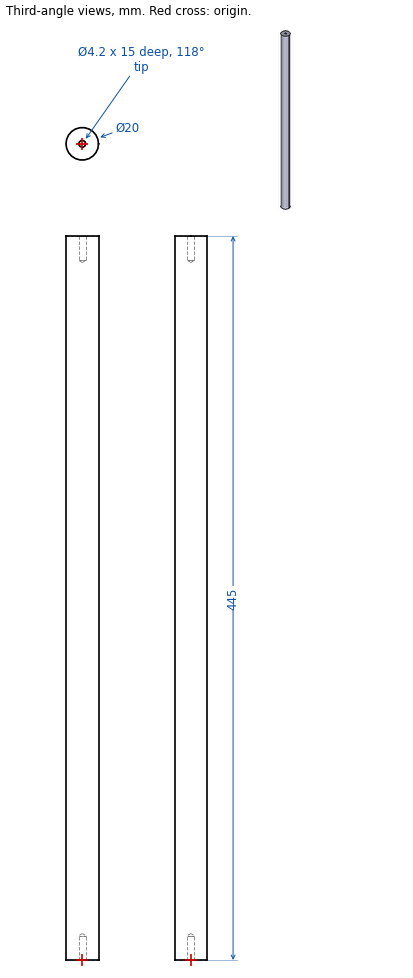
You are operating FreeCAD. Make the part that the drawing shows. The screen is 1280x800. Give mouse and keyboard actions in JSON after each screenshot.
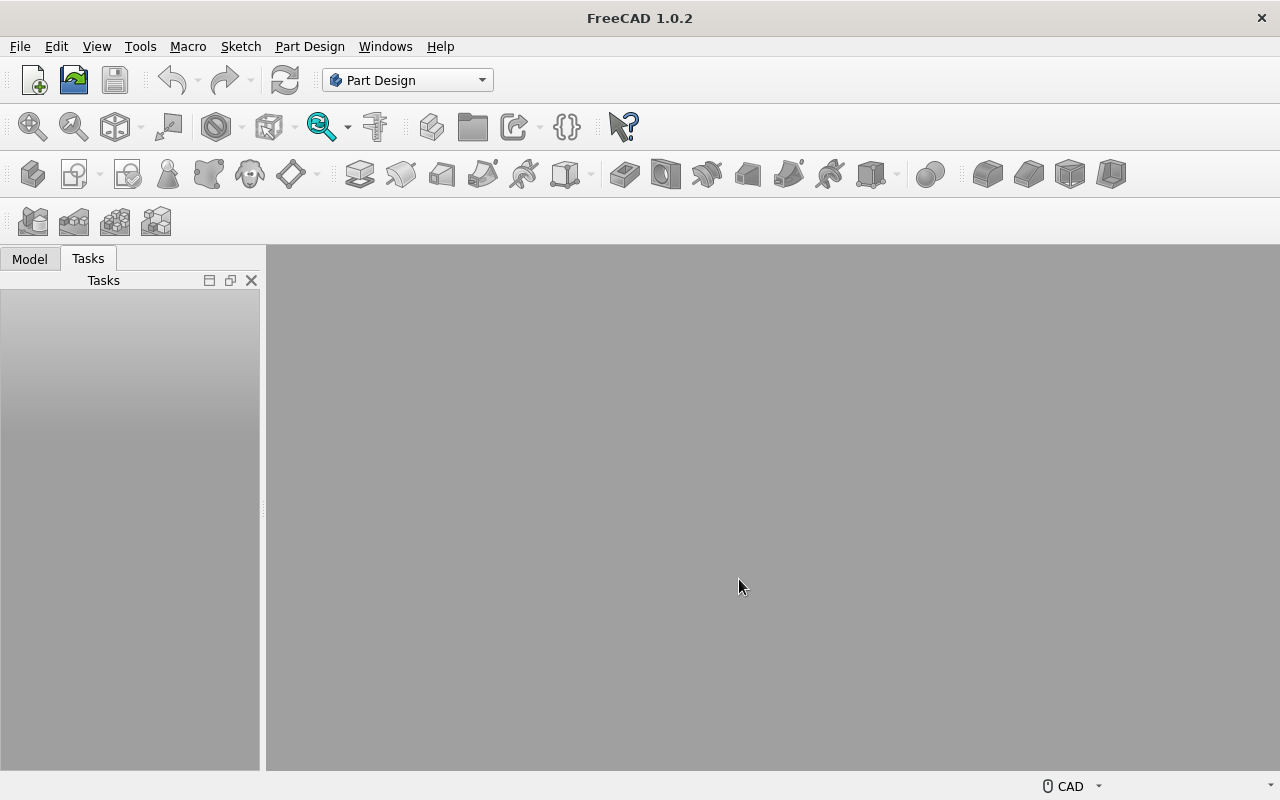
{"action": "key", "text": "ctrl+n"}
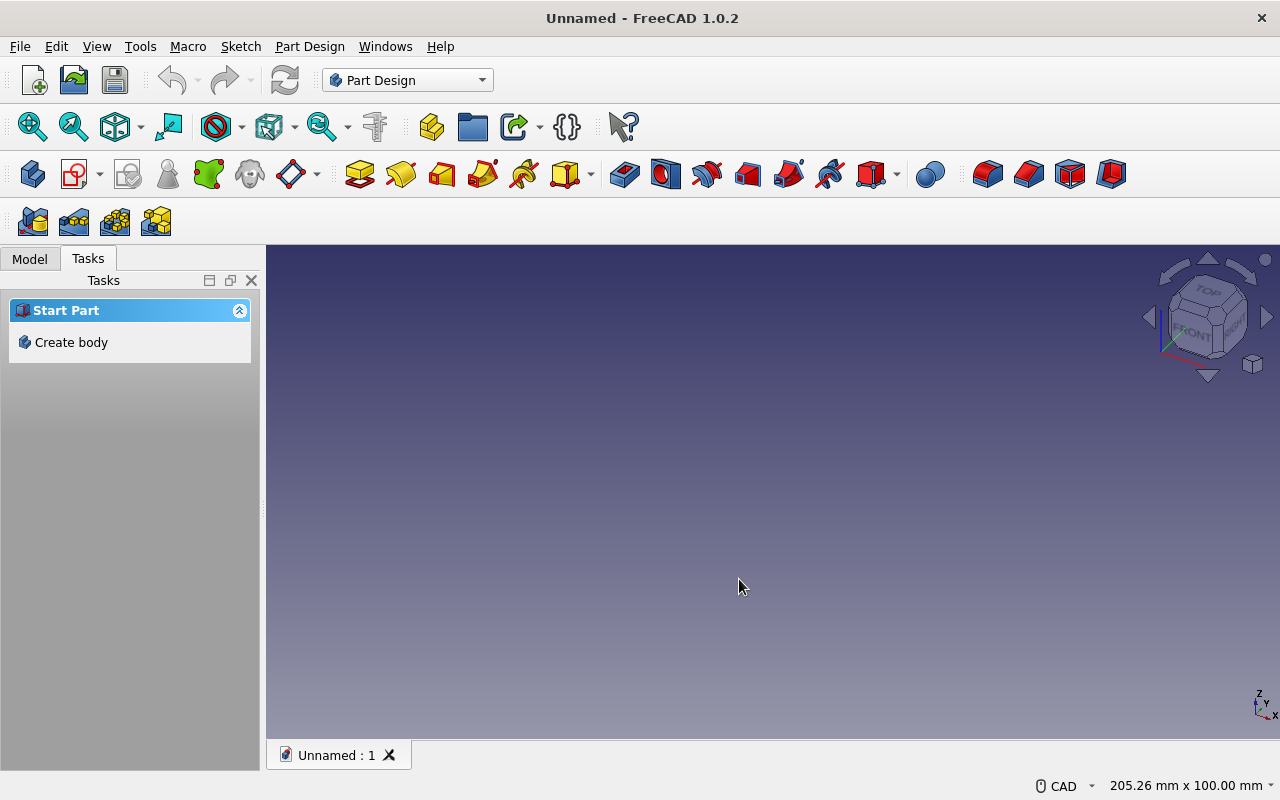
{"action": "left_click", "coordinate": [74, 174]}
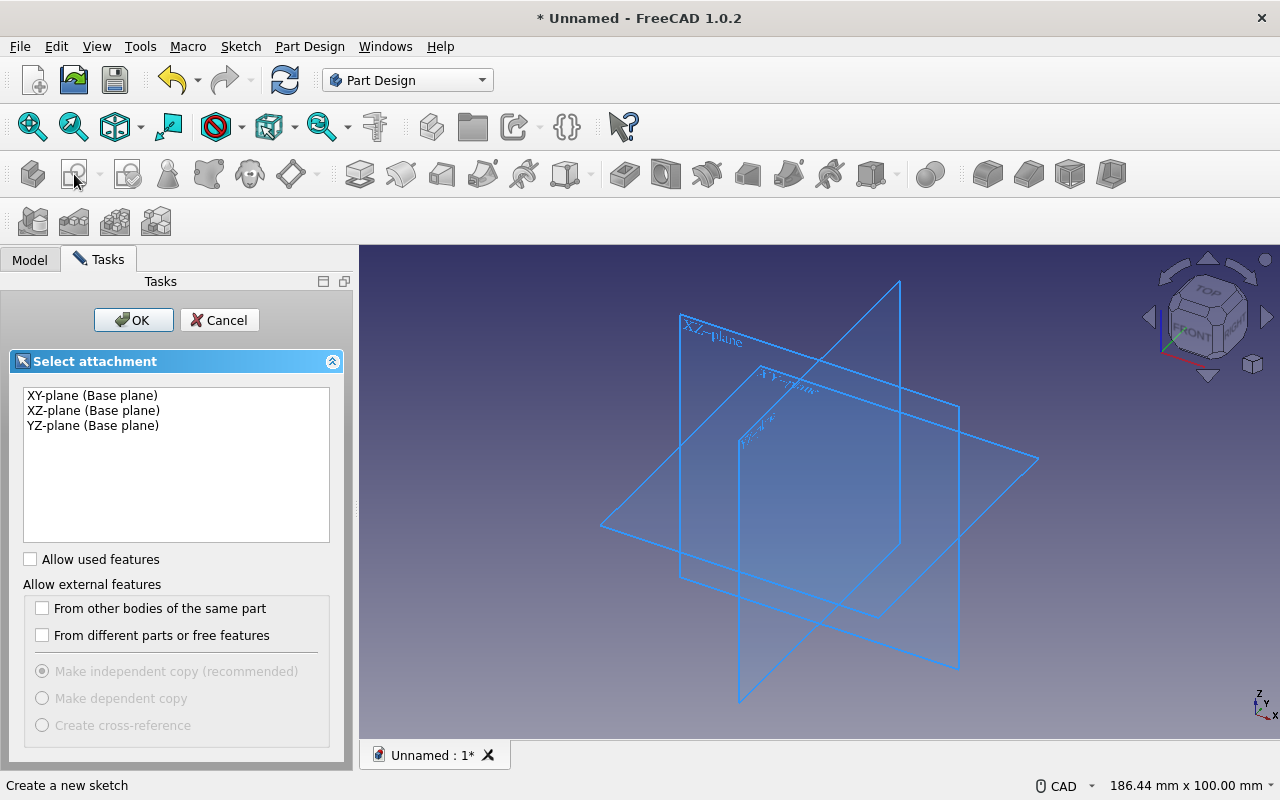
{"action": "left_click", "coordinate": [84, 396]}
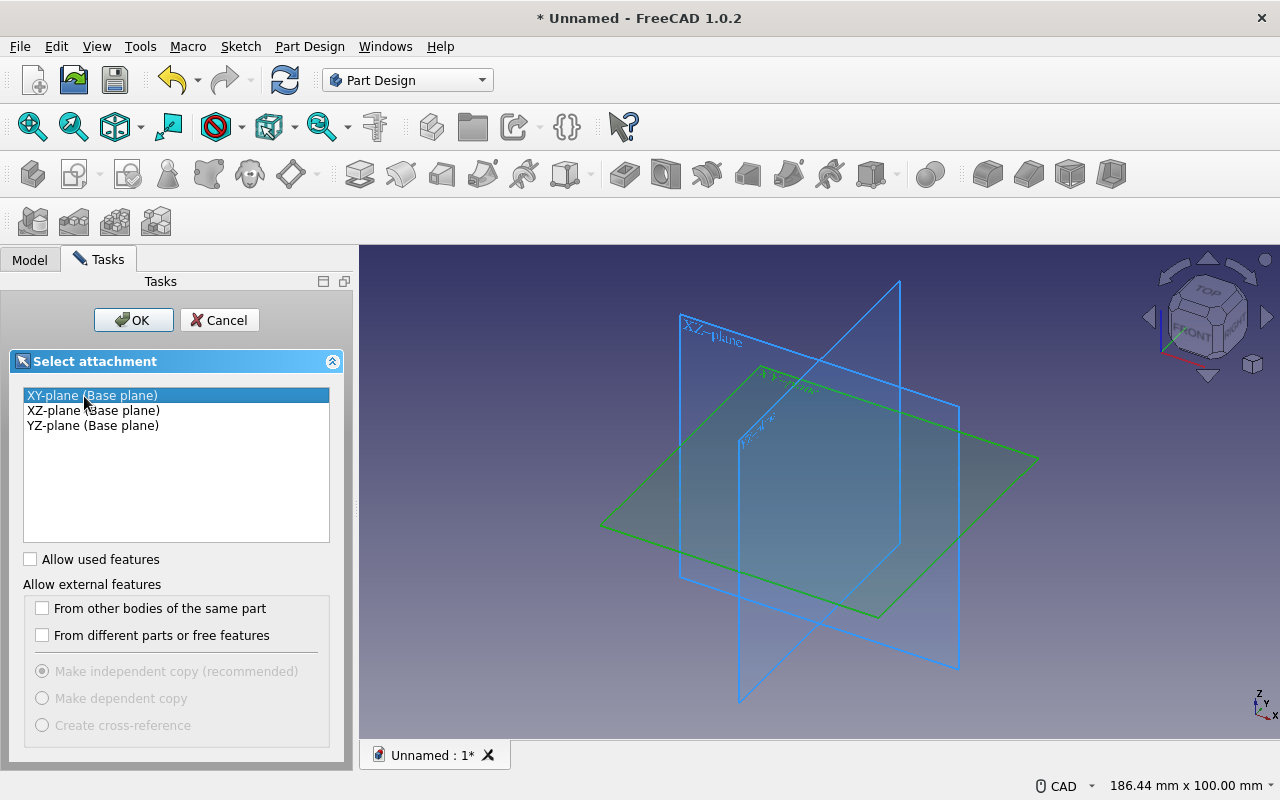
{"action": "left_click", "coordinate": [134, 320]}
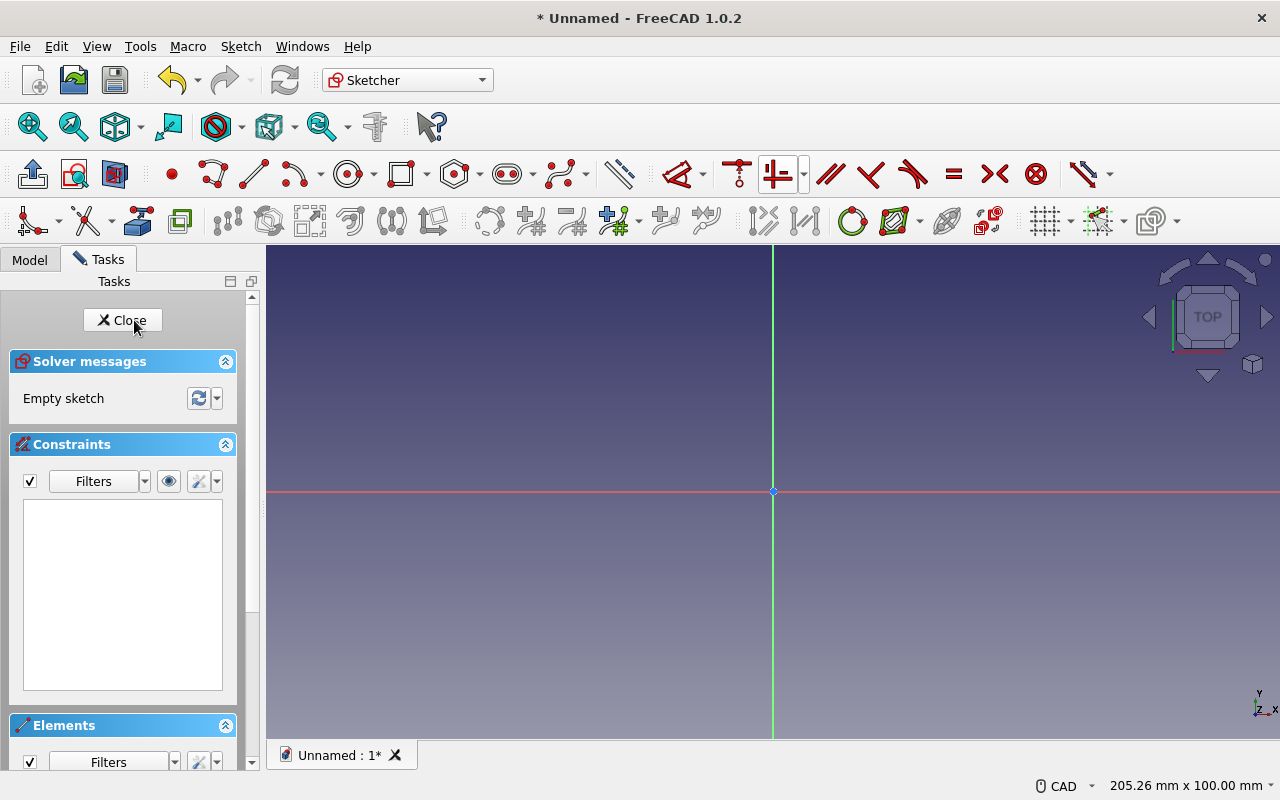
{"action": "scroll", "coordinate": [803, 492], "scroll_direction": "up", "scroll_amount": 6}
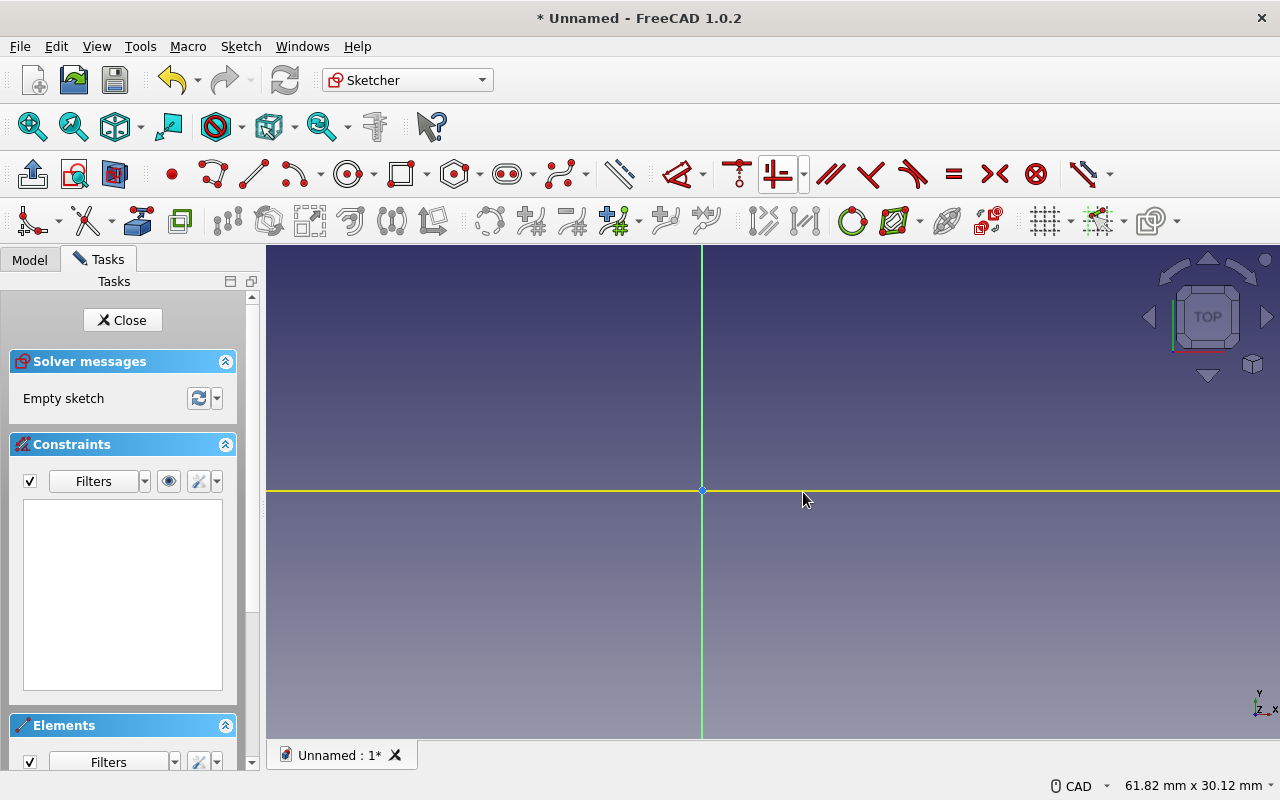
{"action": "key", "text": "g c"}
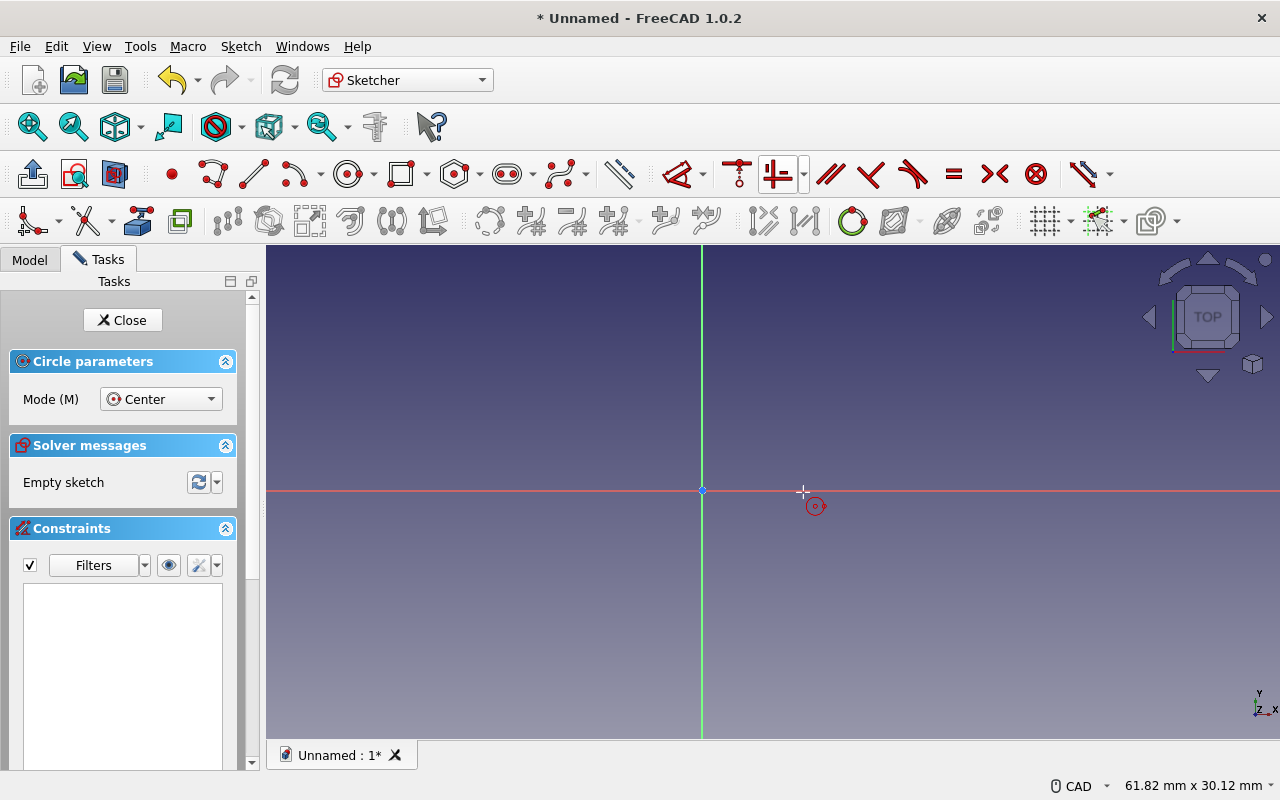
{"action": "left_click", "coordinate": [702, 491]}
{"action": "left_click", "coordinate": [818, 375]}
{"action": "key", "text": "Escape"}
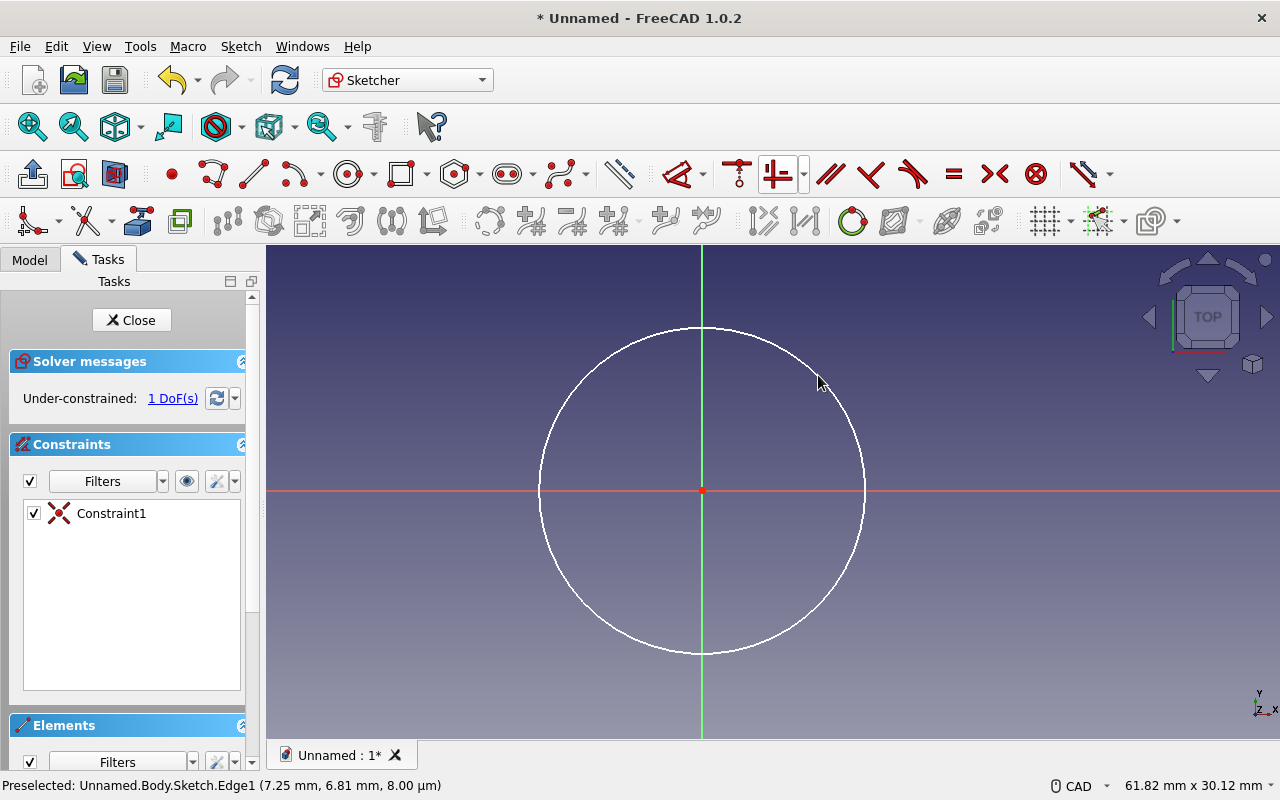
{"action": "left_click", "coordinate": [817, 375]}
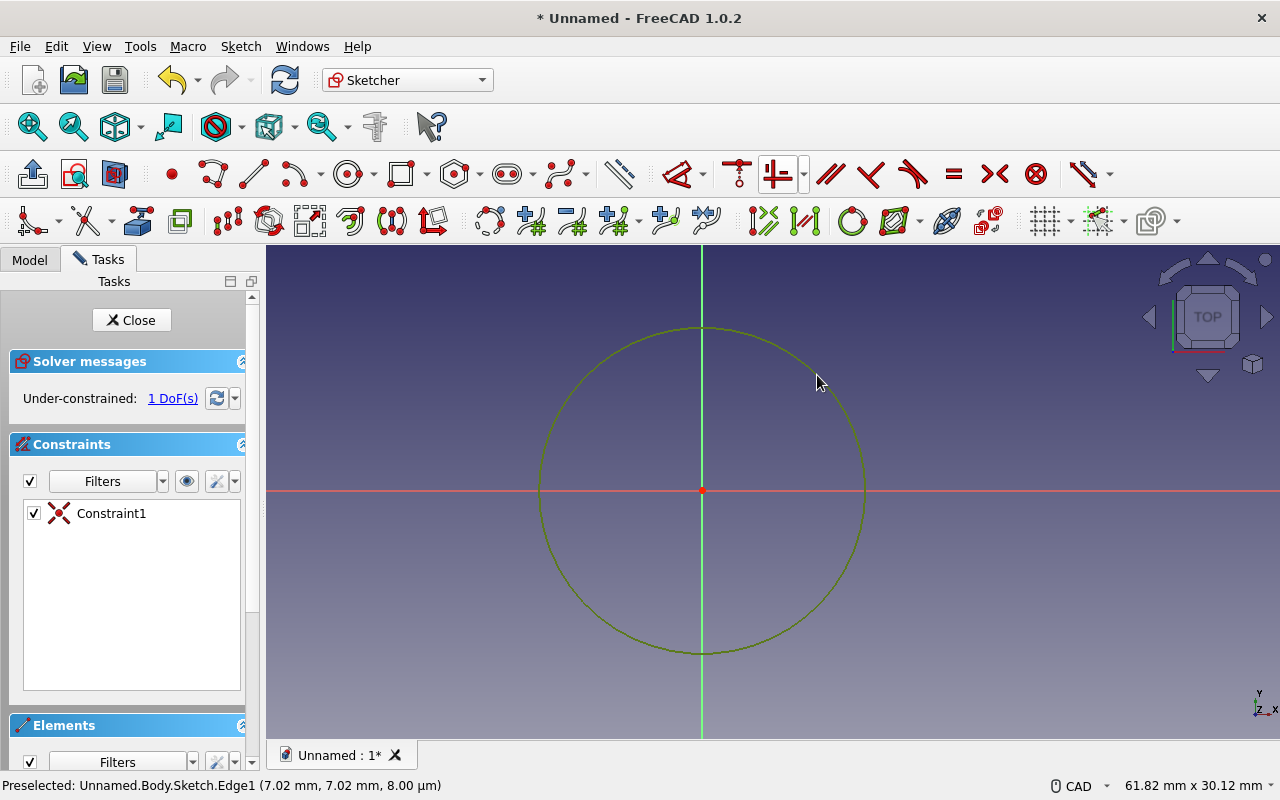
{"action": "key", "text": "k o"}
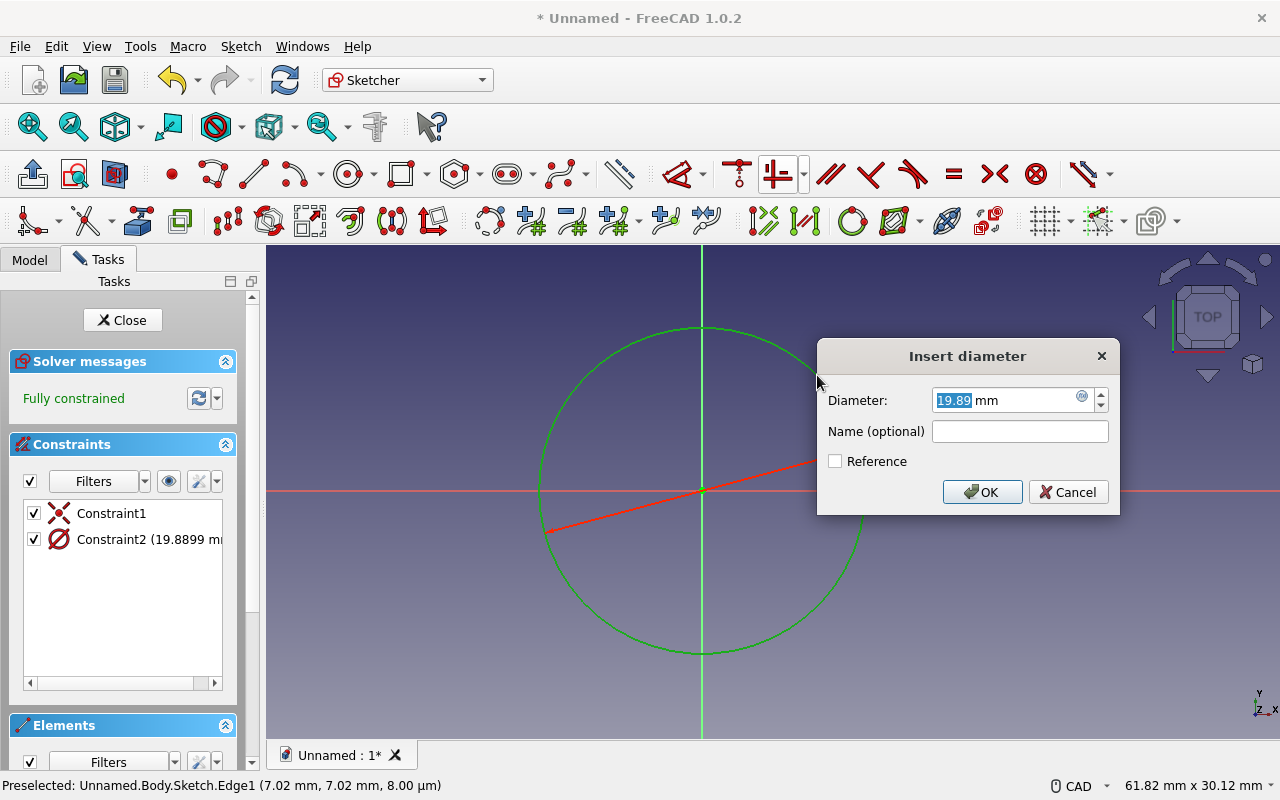
{"action": "type", "text": "20"}
{"action": "key", "text": "Return"}